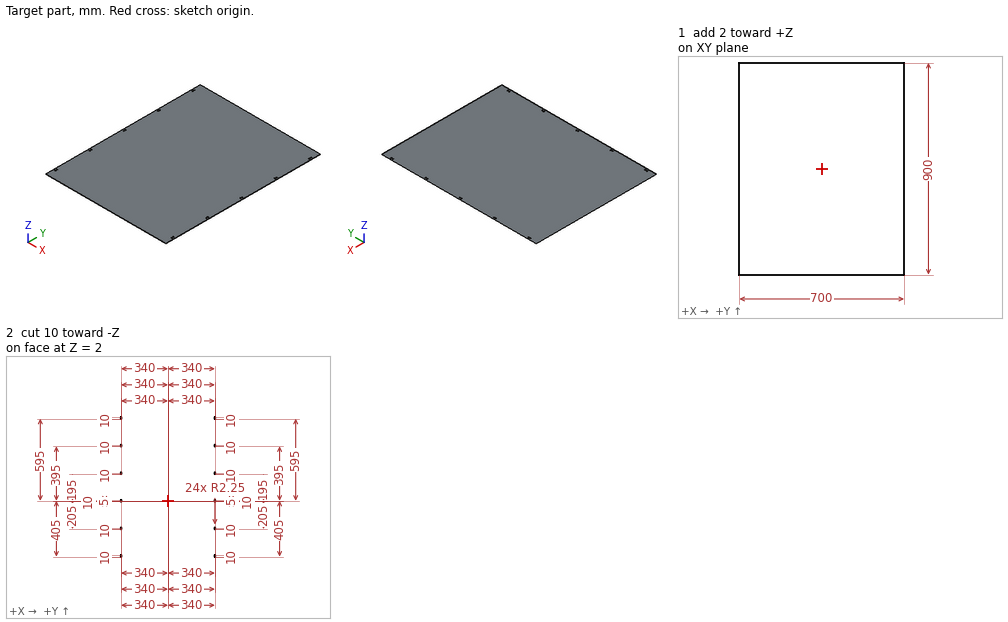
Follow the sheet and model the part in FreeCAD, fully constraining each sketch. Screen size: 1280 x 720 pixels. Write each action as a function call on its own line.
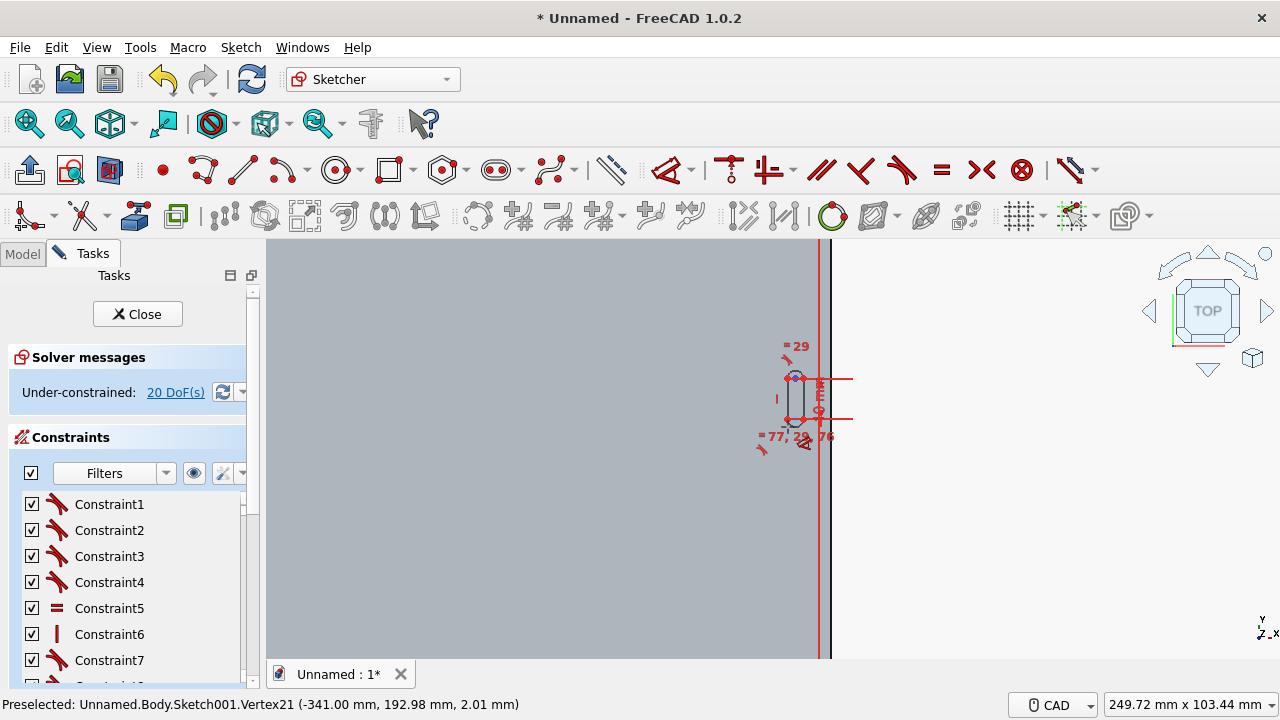
click(788, 419)
click(822, 525)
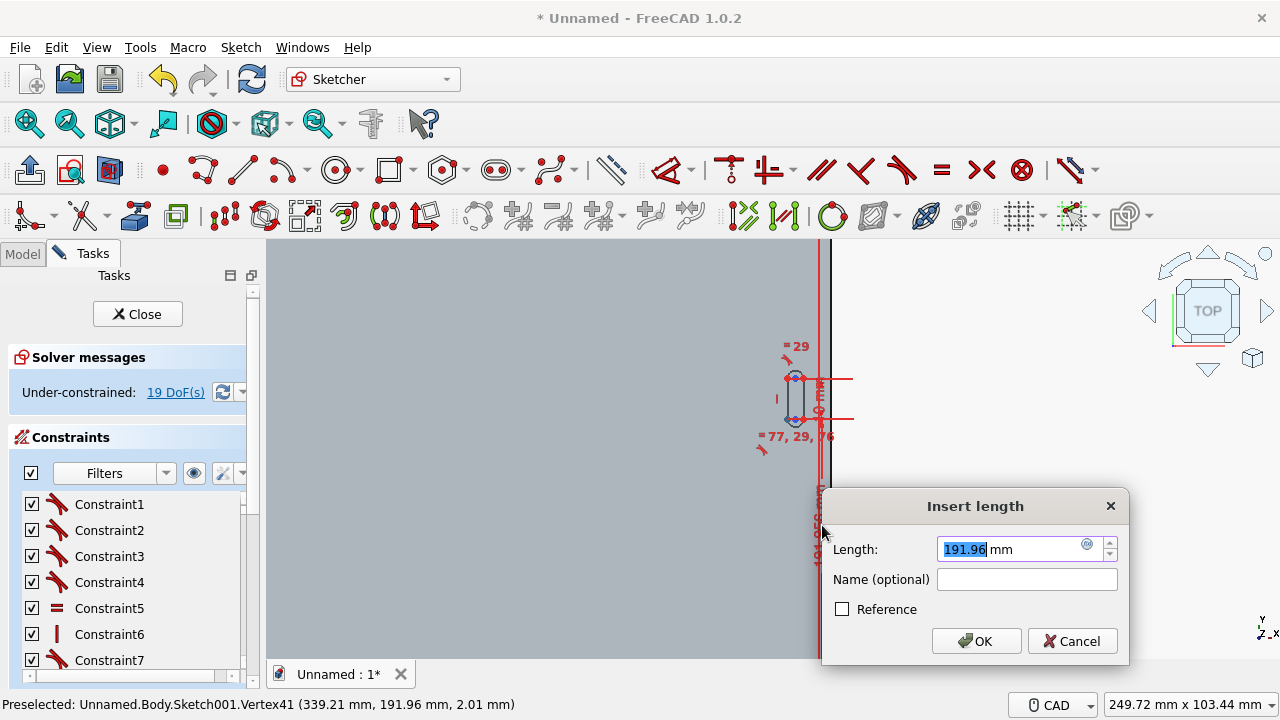
text(195)
key(Return)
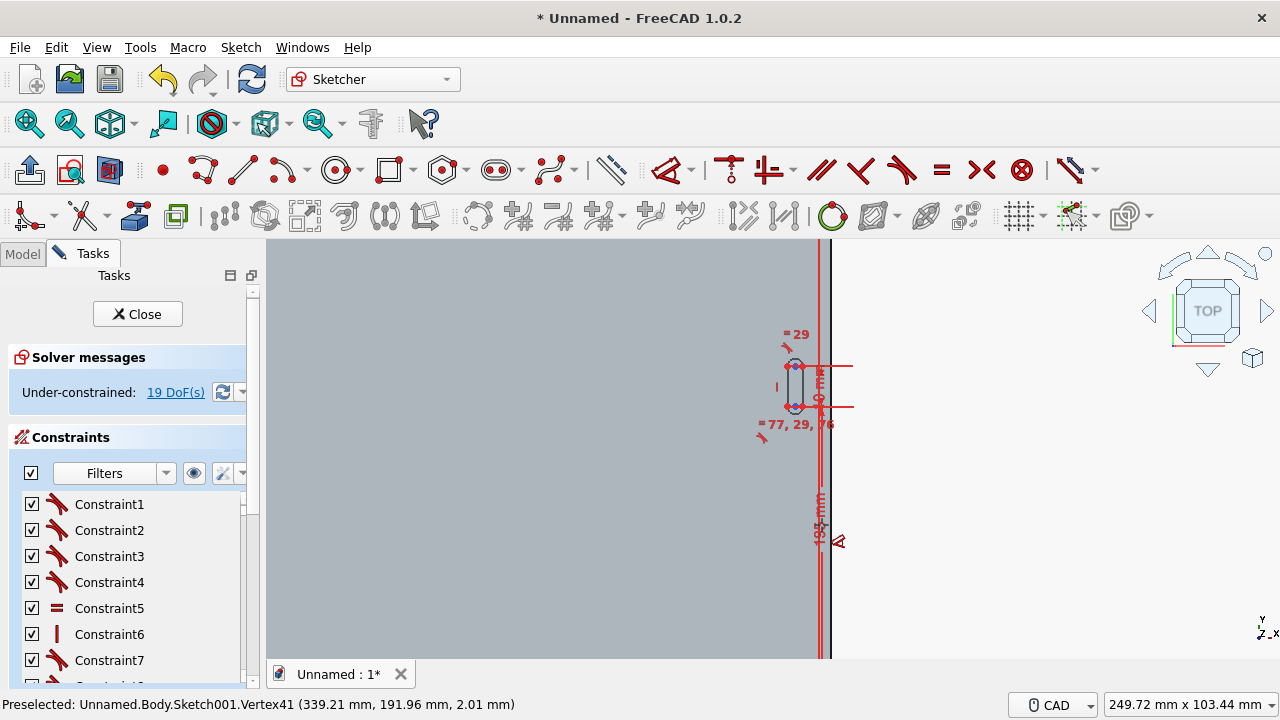
scroll(788, 427, down, 14)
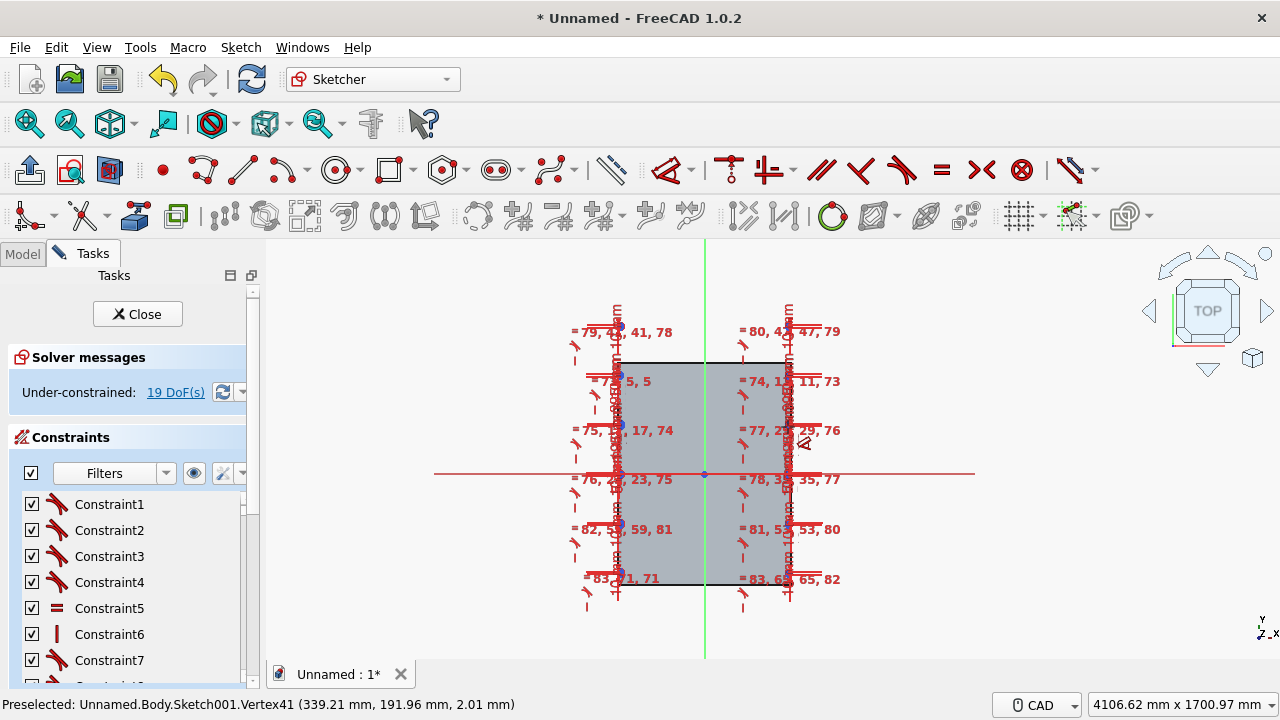
scroll(620, 328, up, 14)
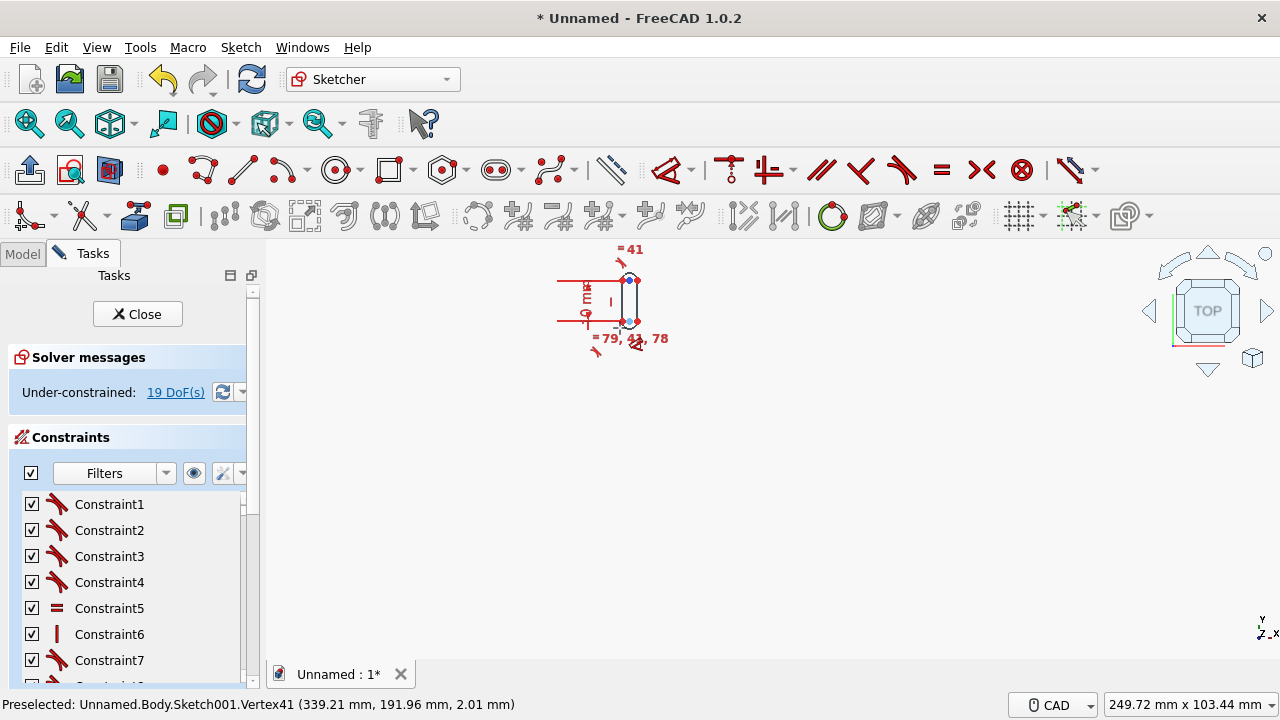
click(622, 321)
click(588, 476)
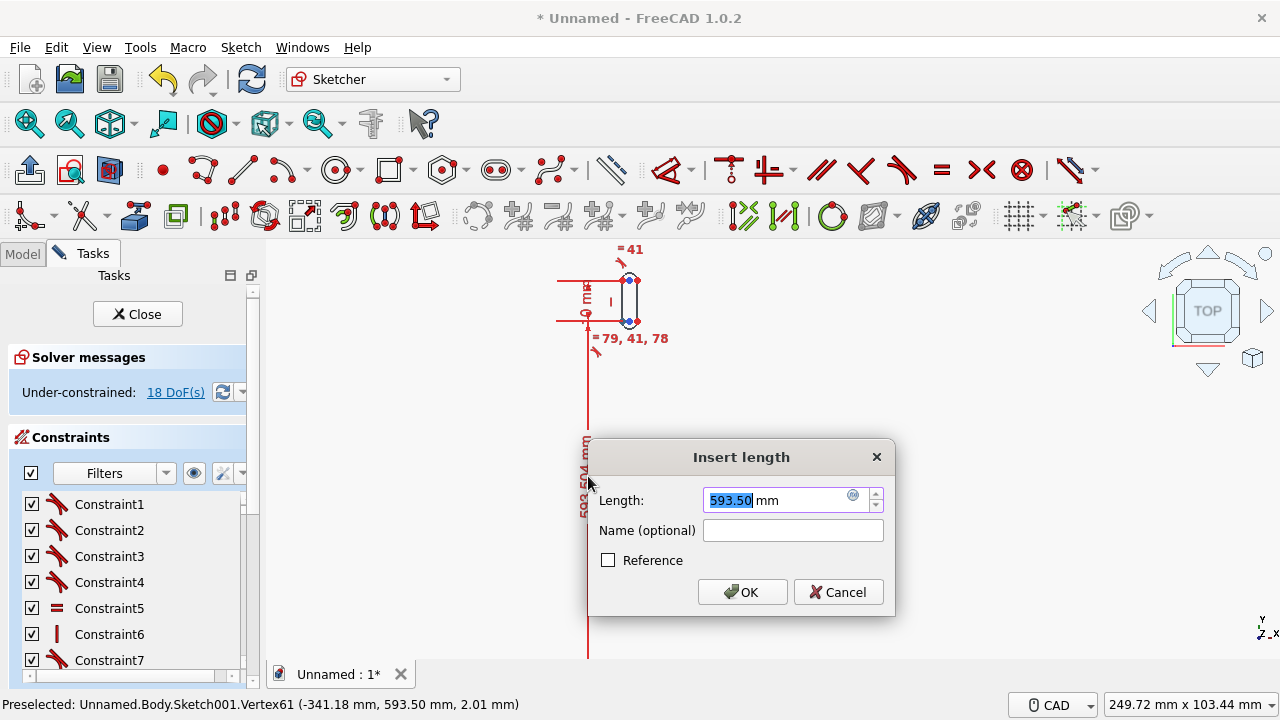
text(595)
key(Return)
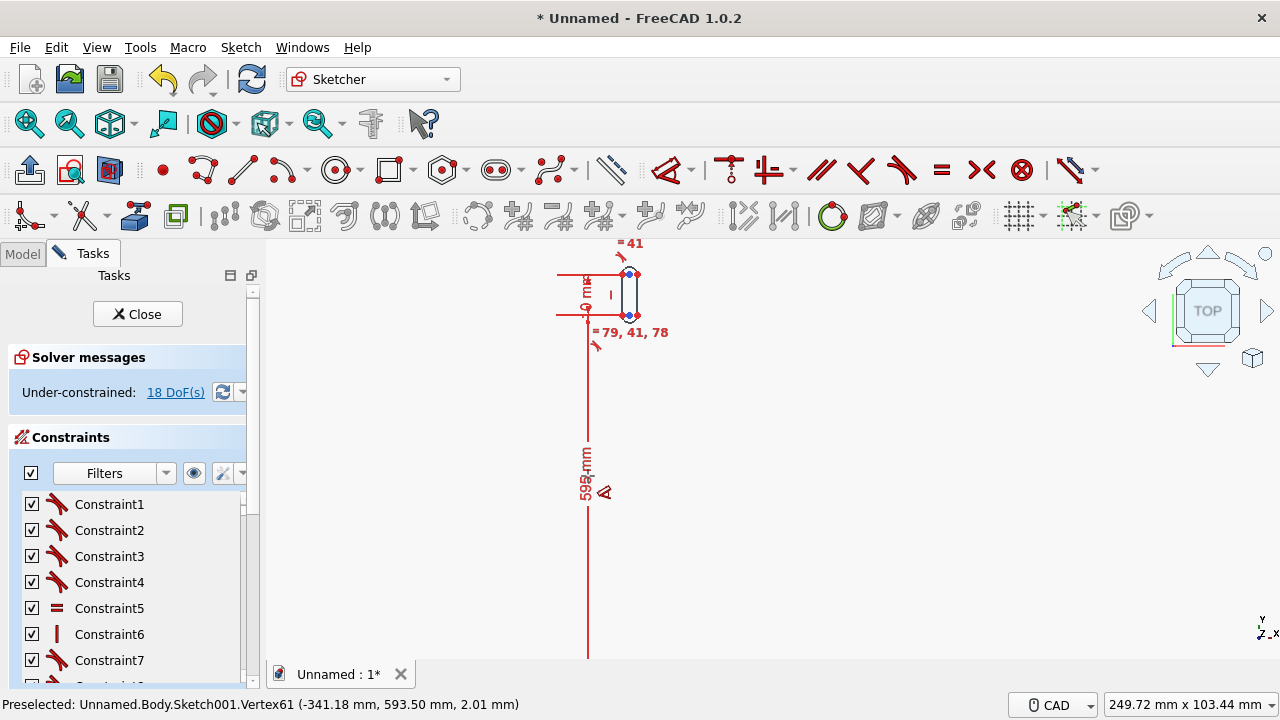
scroll(620, 328, down, 14)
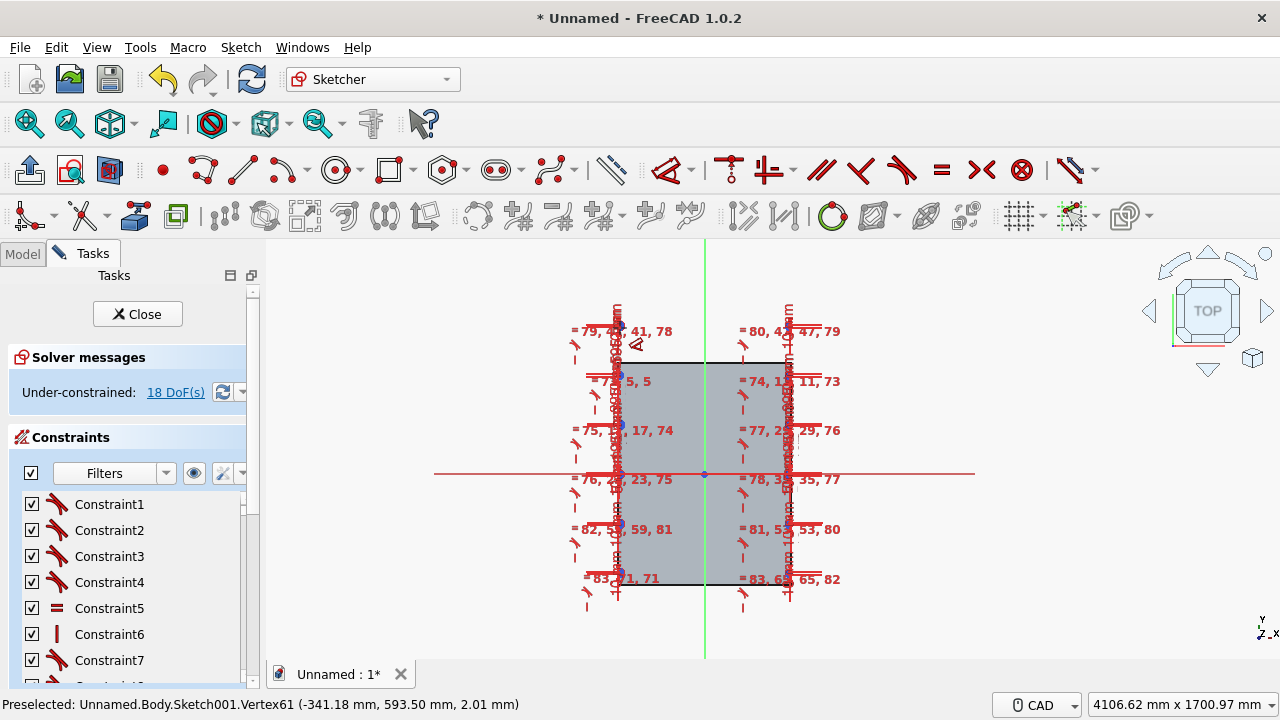
scroll(788, 328, up, 14)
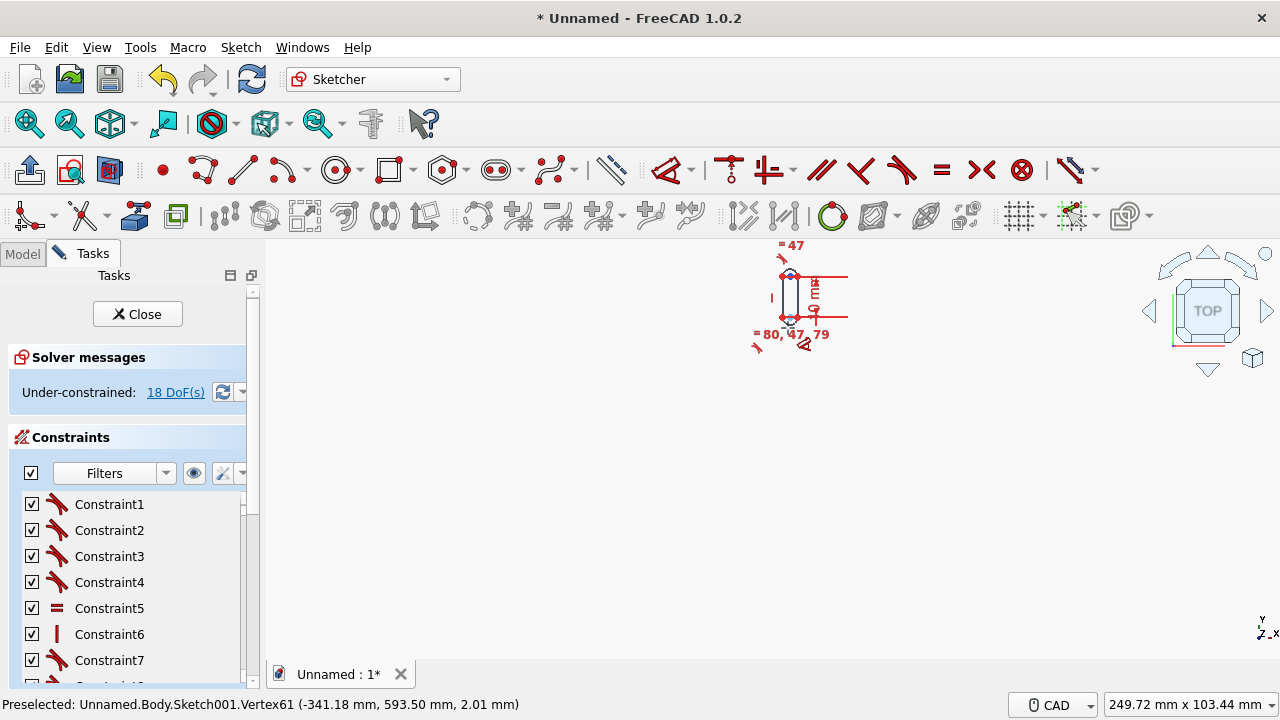
click(783, 317)
click(817, 474)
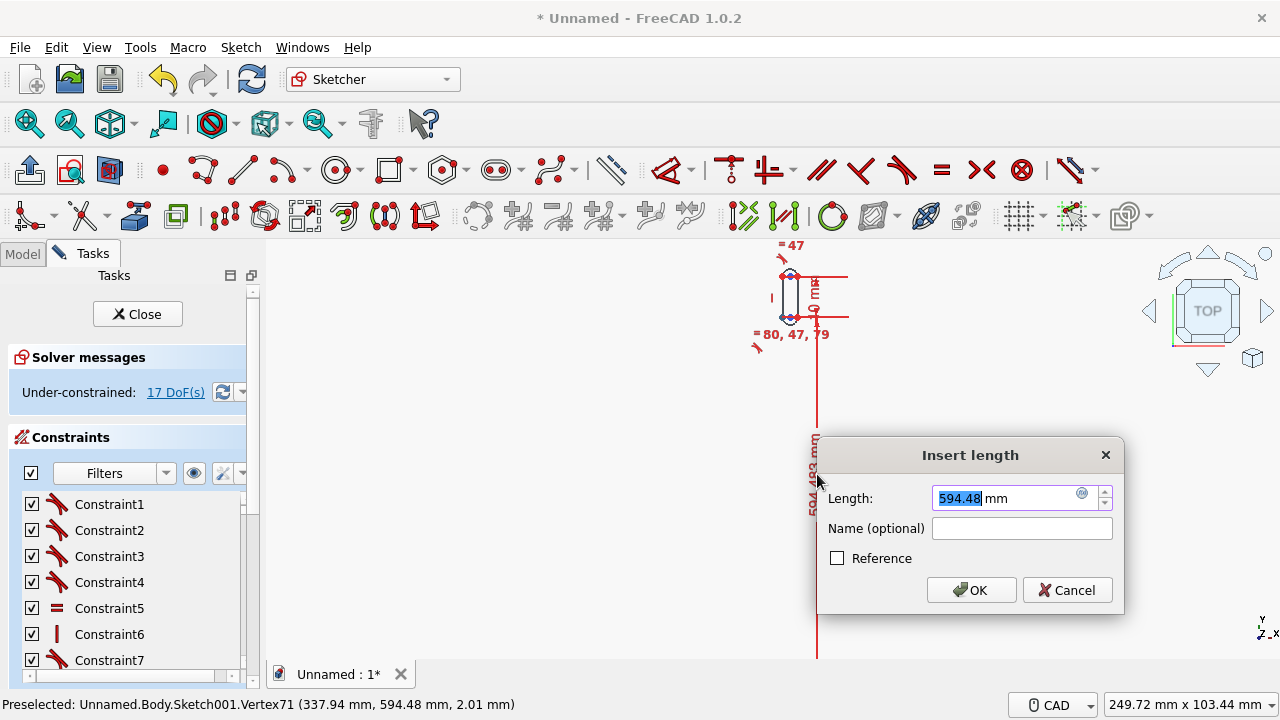
text(595)
key(Return)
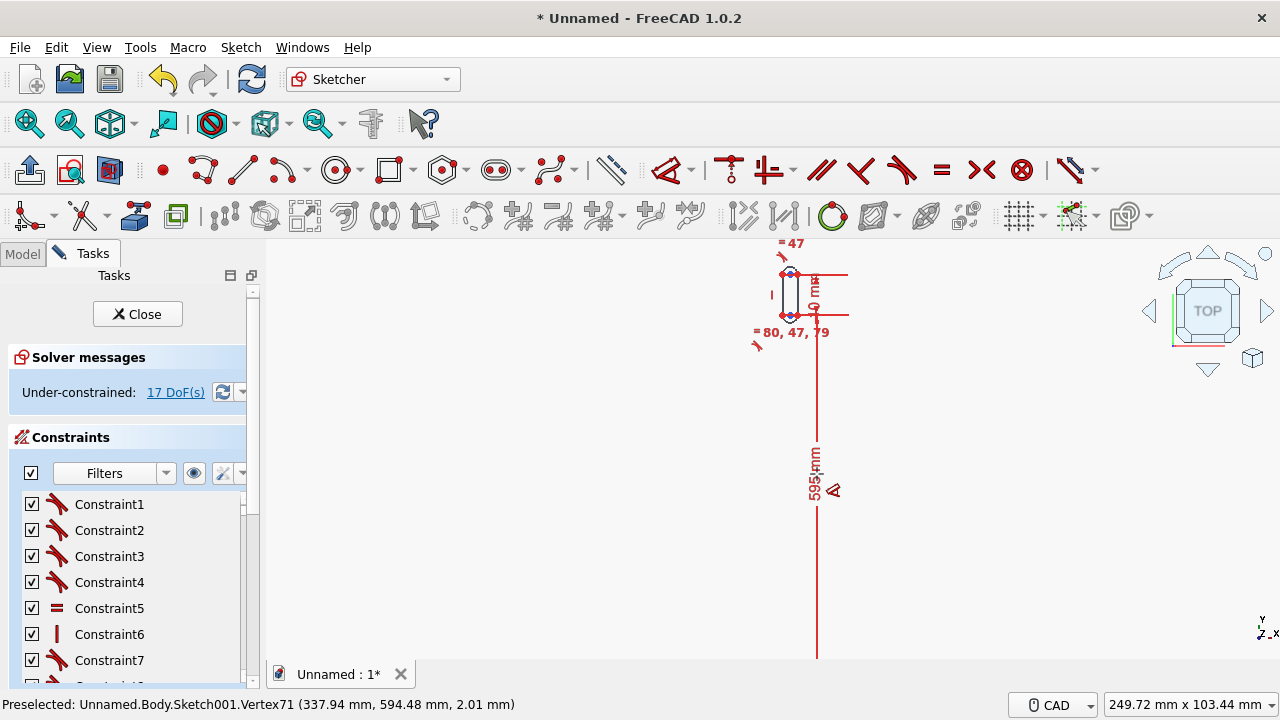
scroll(788, 328, down, 14)